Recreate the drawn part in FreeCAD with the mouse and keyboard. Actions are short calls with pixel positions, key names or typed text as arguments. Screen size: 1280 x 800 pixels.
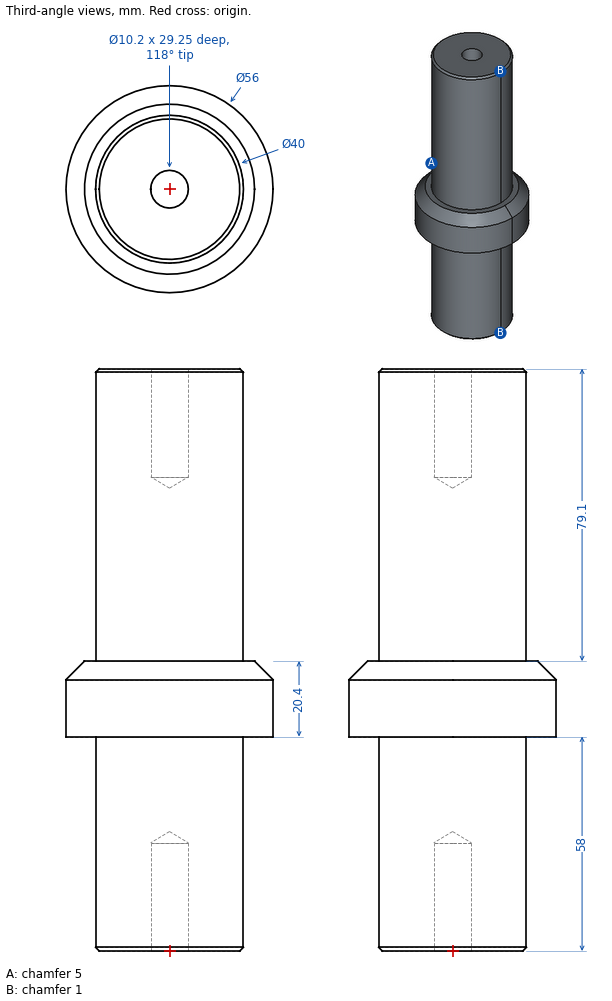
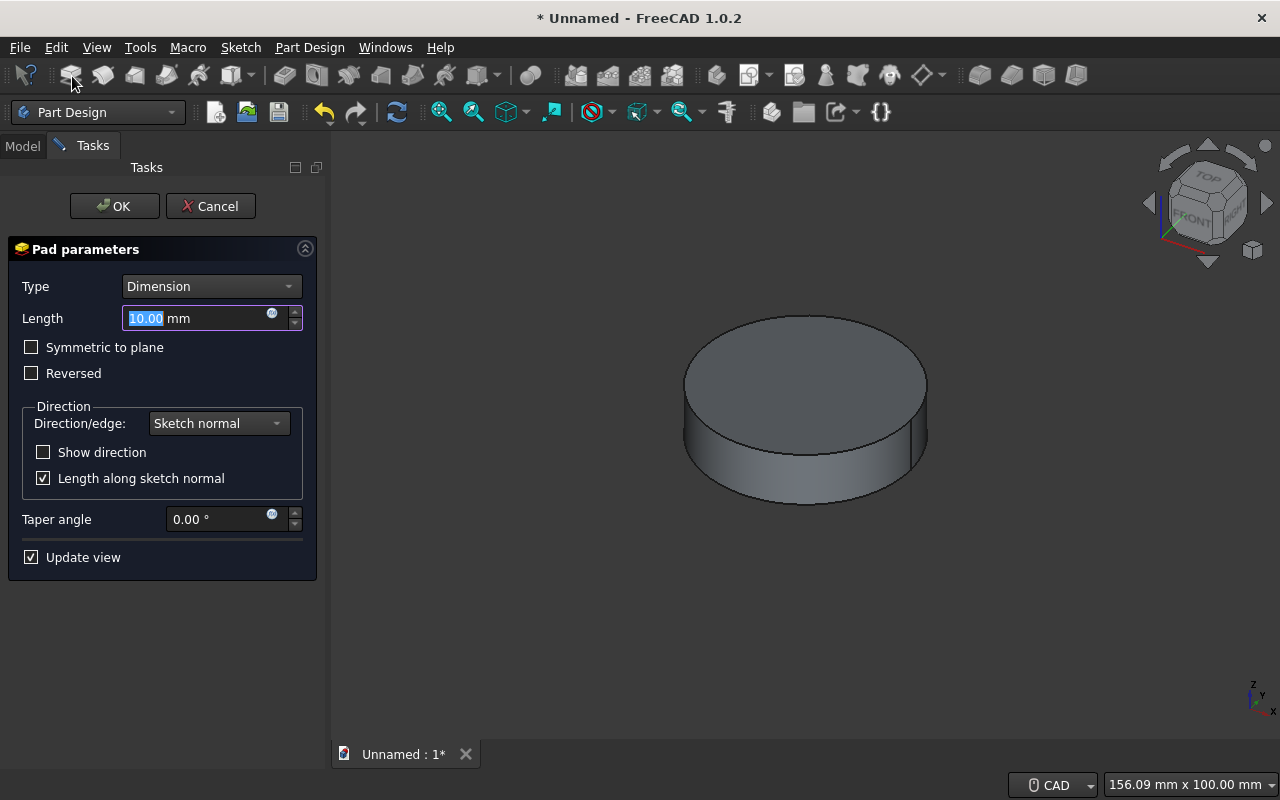
text(58)
key(Tab)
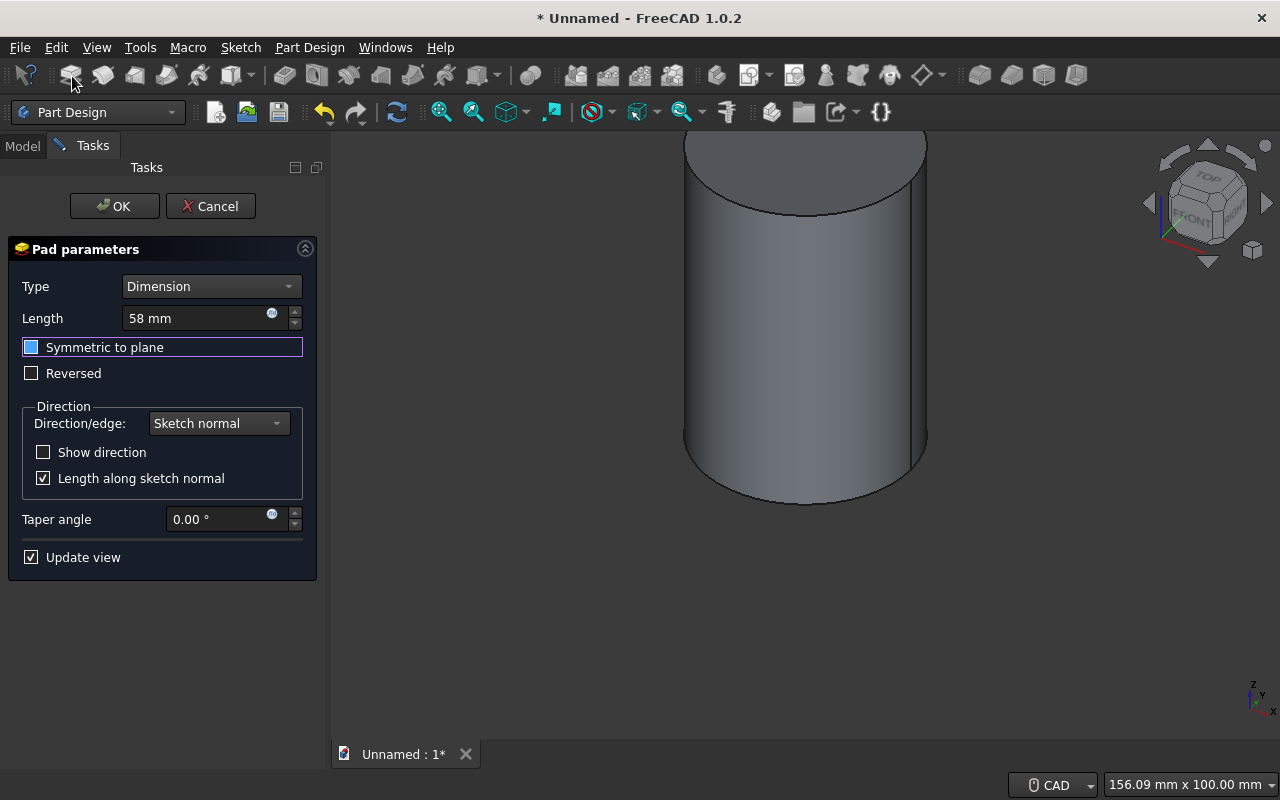
click(115, 206)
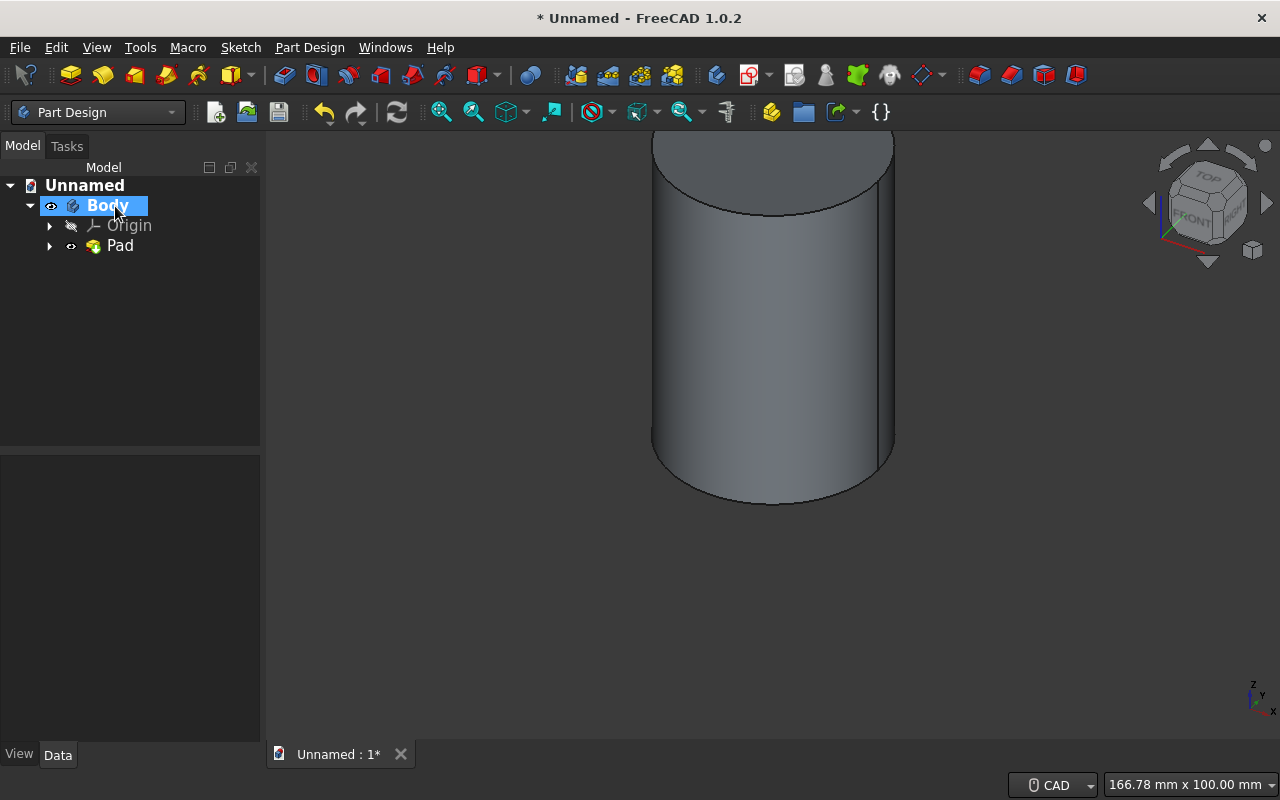
click(442, 112)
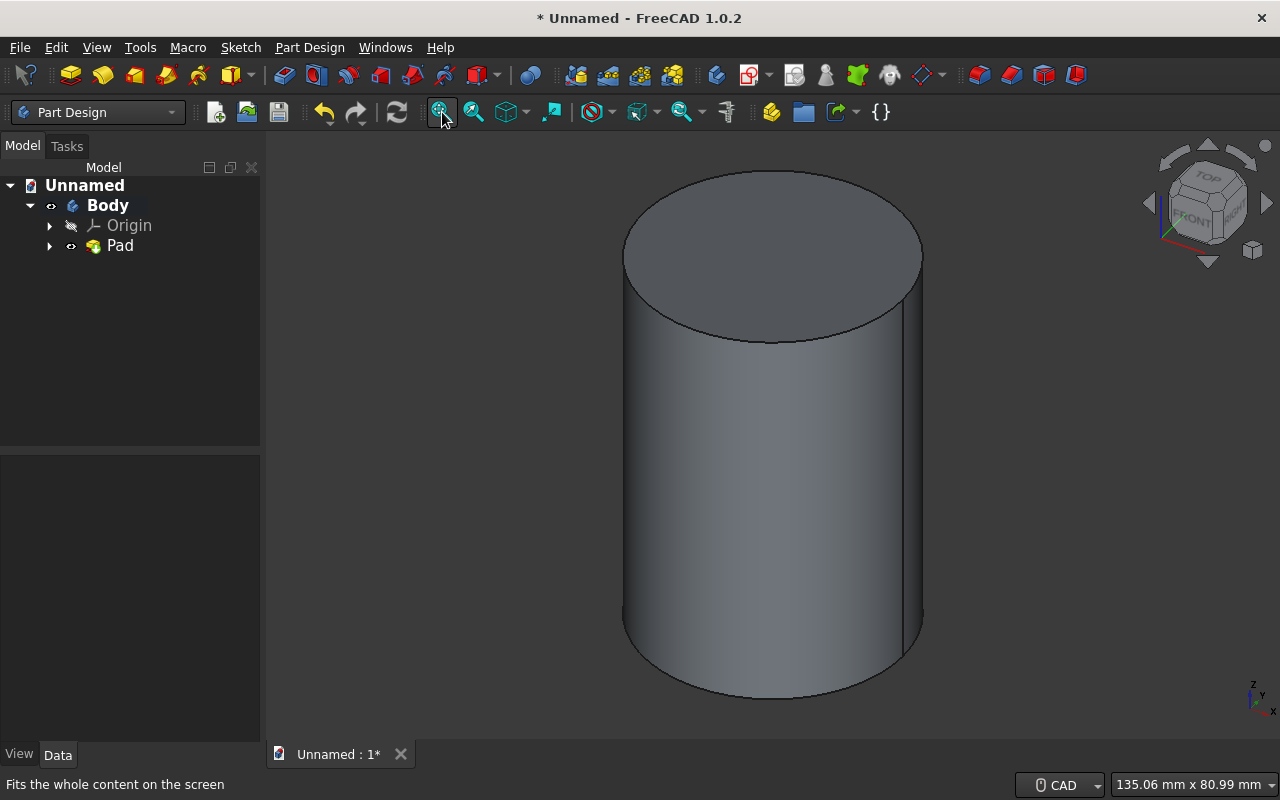
click(773, 256)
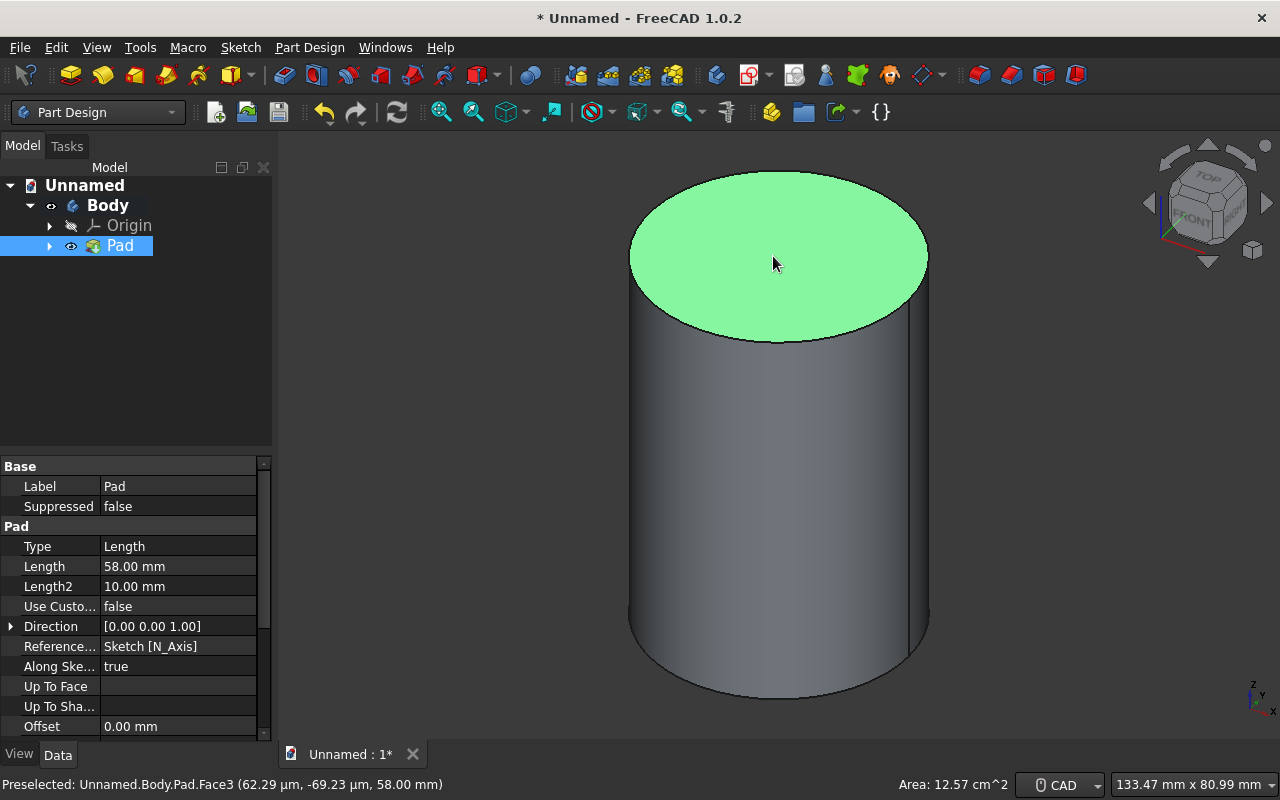
click(750, 76)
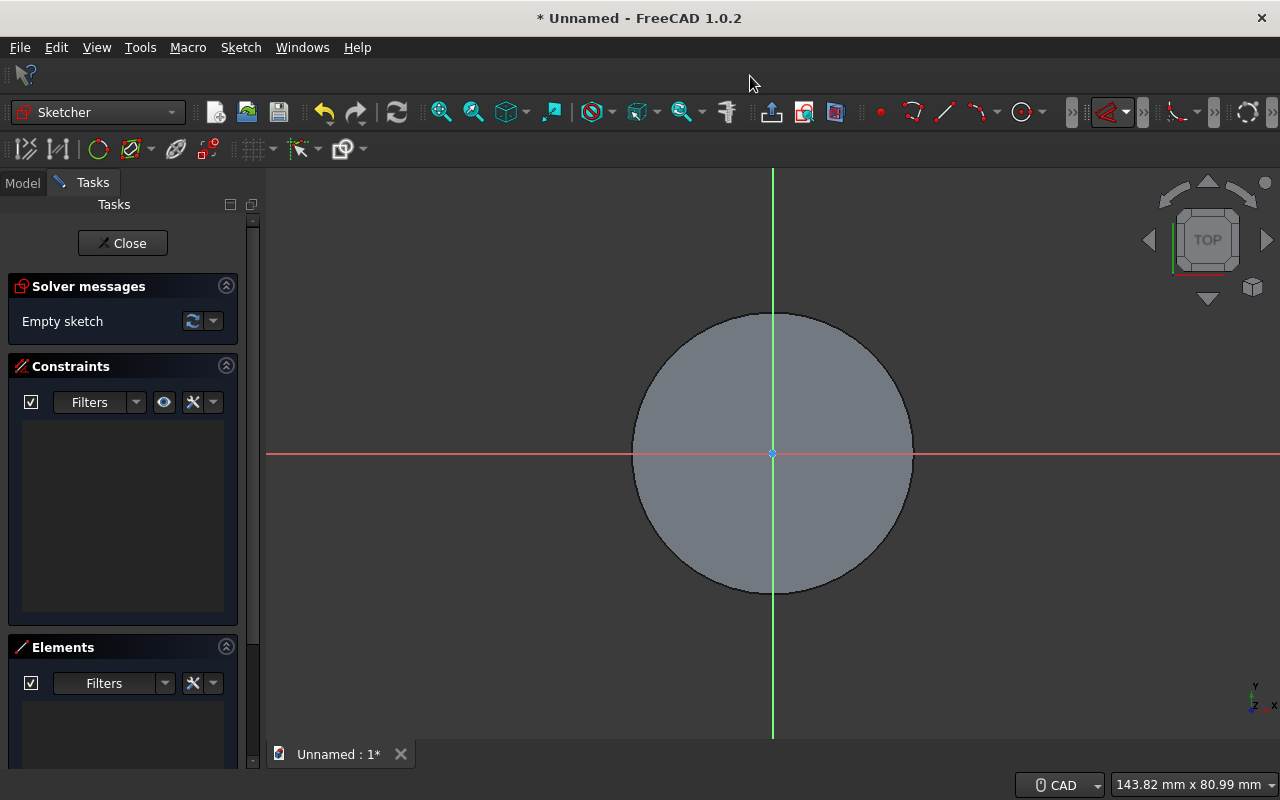
click(1022, 112)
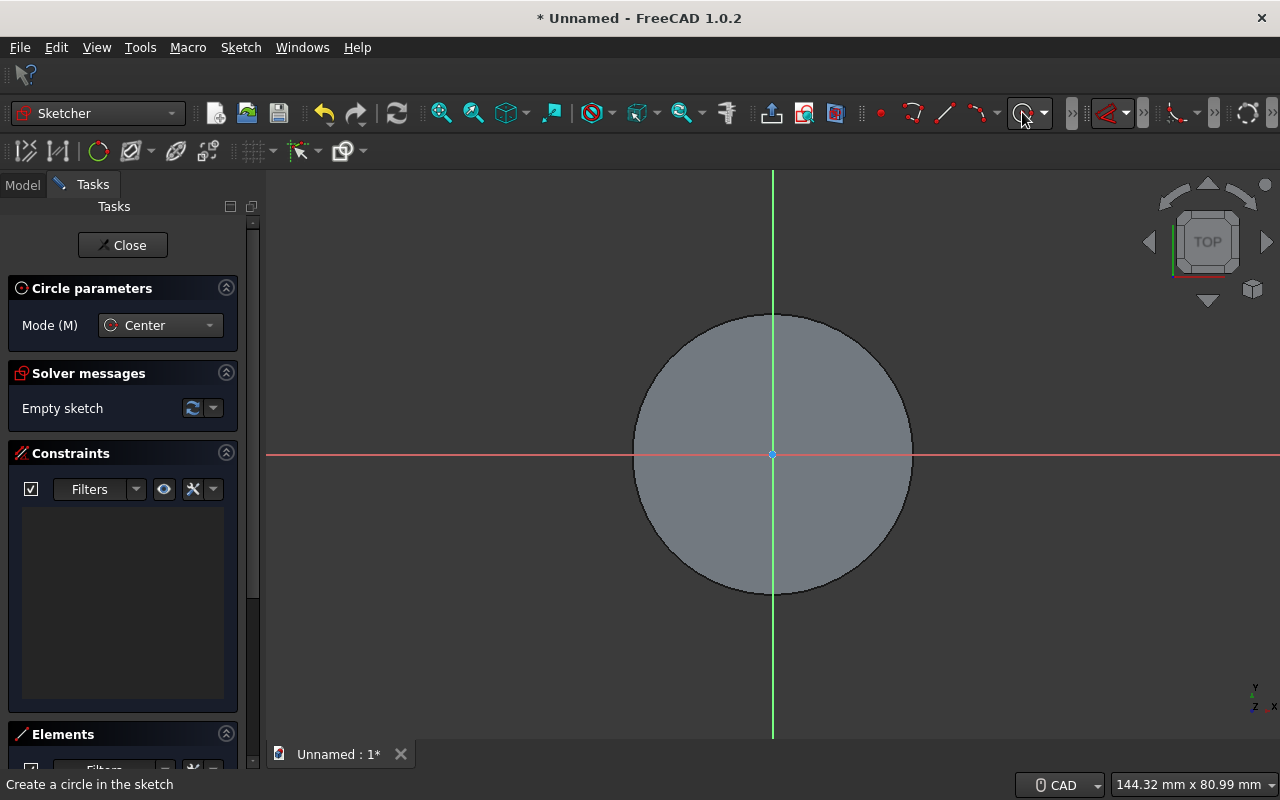
click(773, 454)
move(912, 315)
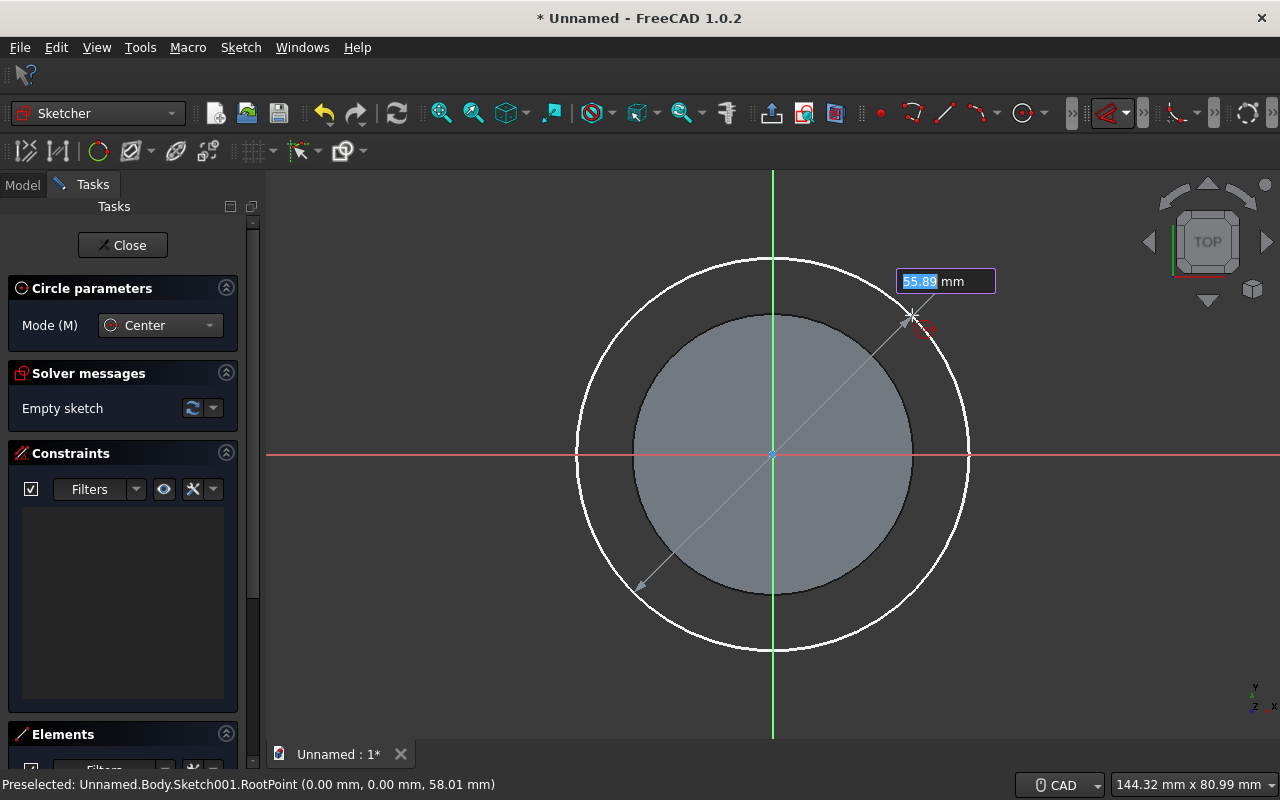
text(56)
key(Return)
key(Escape)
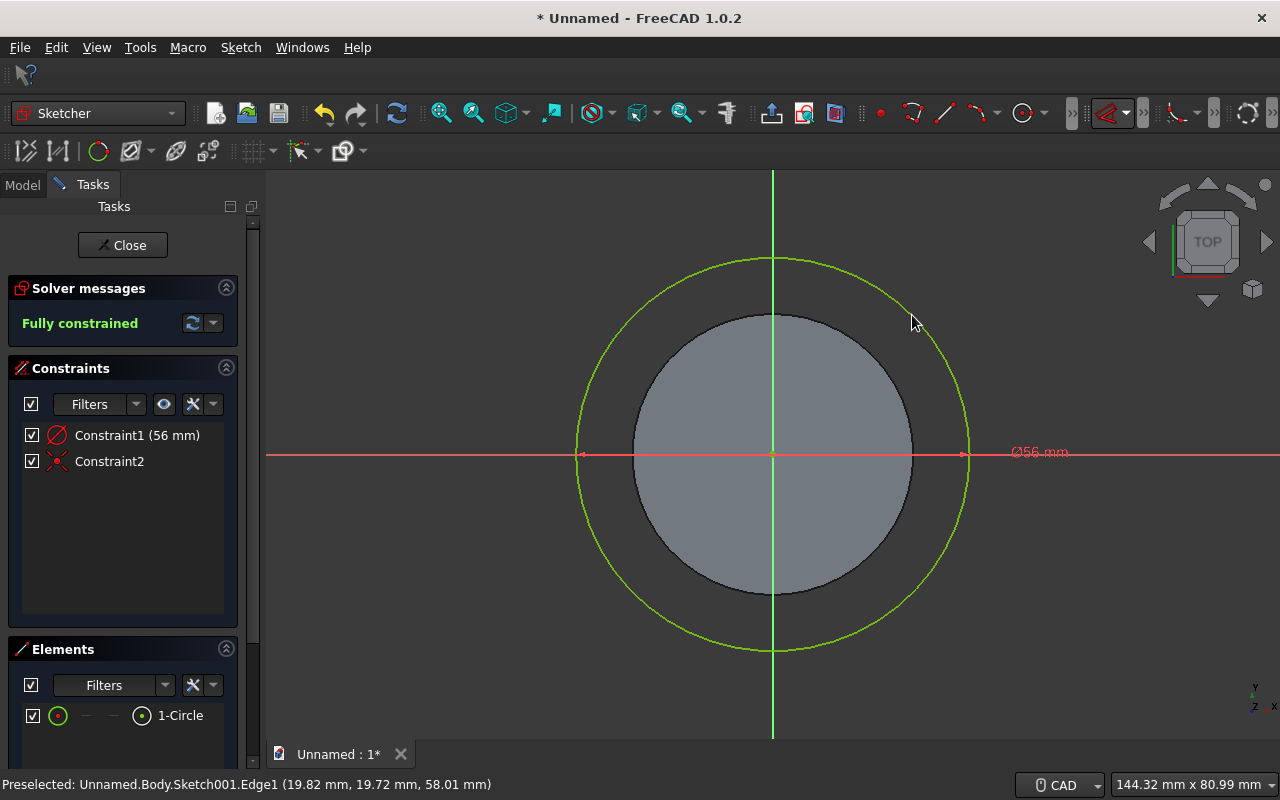
click(123, 245)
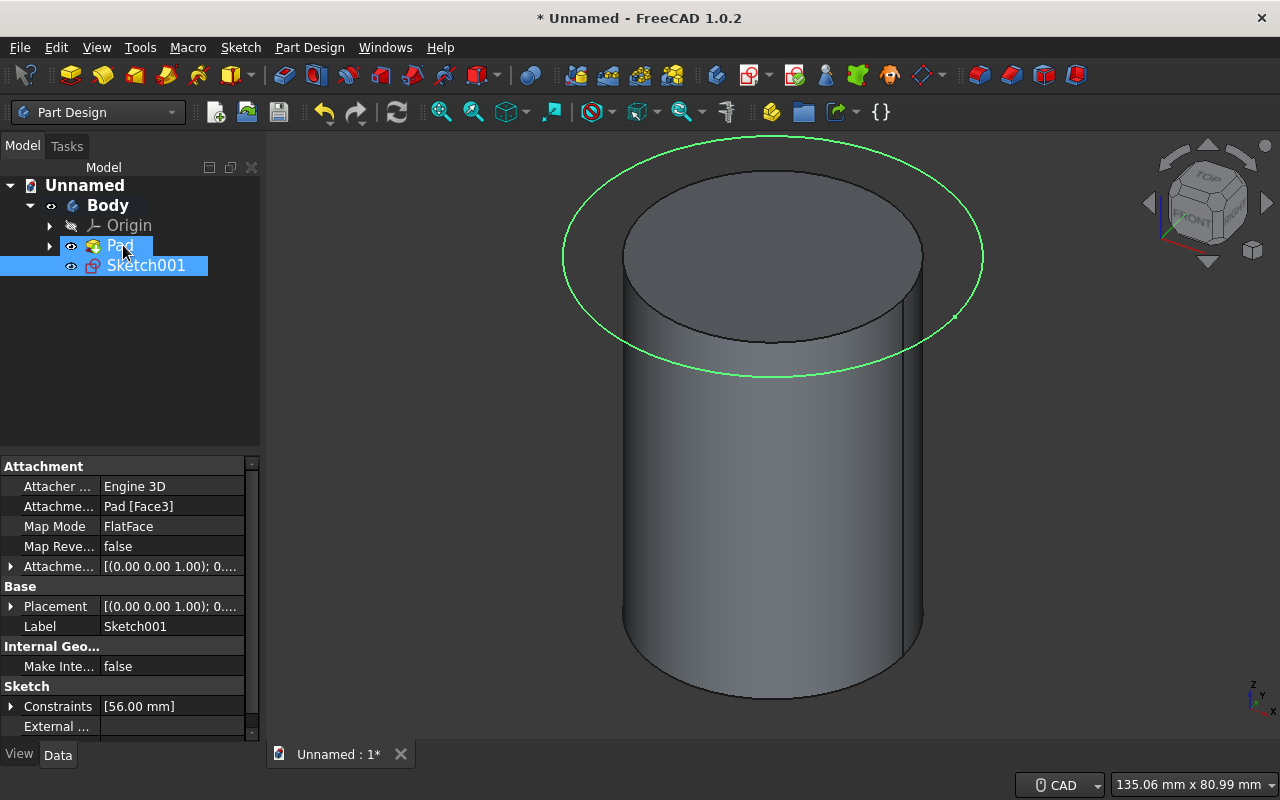
click(72, 76)